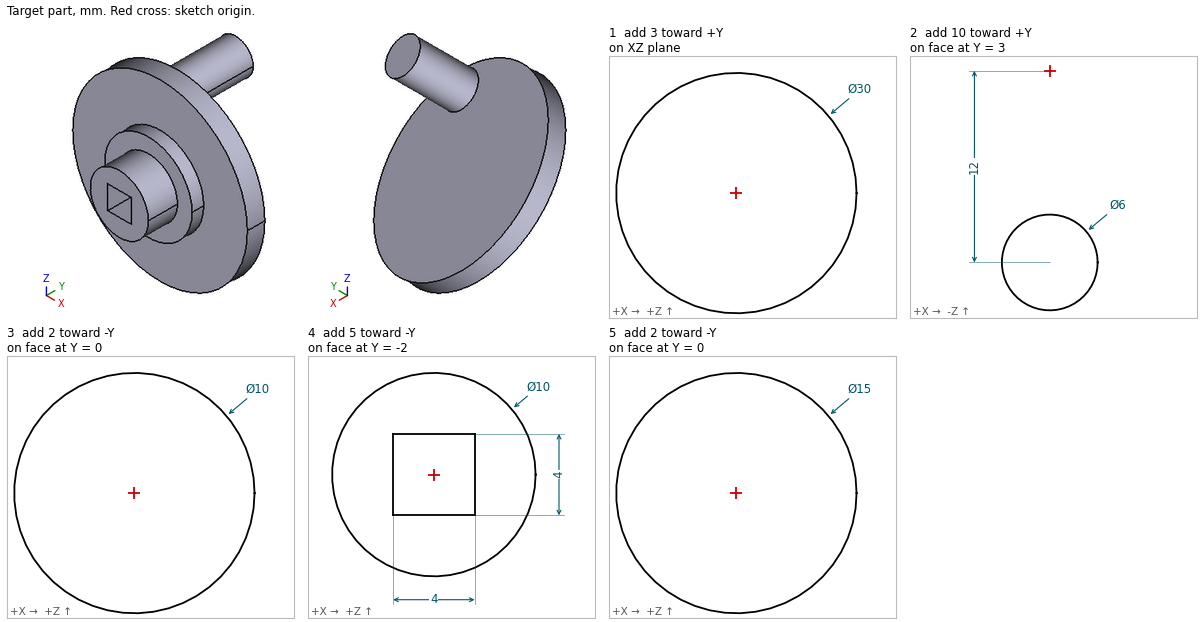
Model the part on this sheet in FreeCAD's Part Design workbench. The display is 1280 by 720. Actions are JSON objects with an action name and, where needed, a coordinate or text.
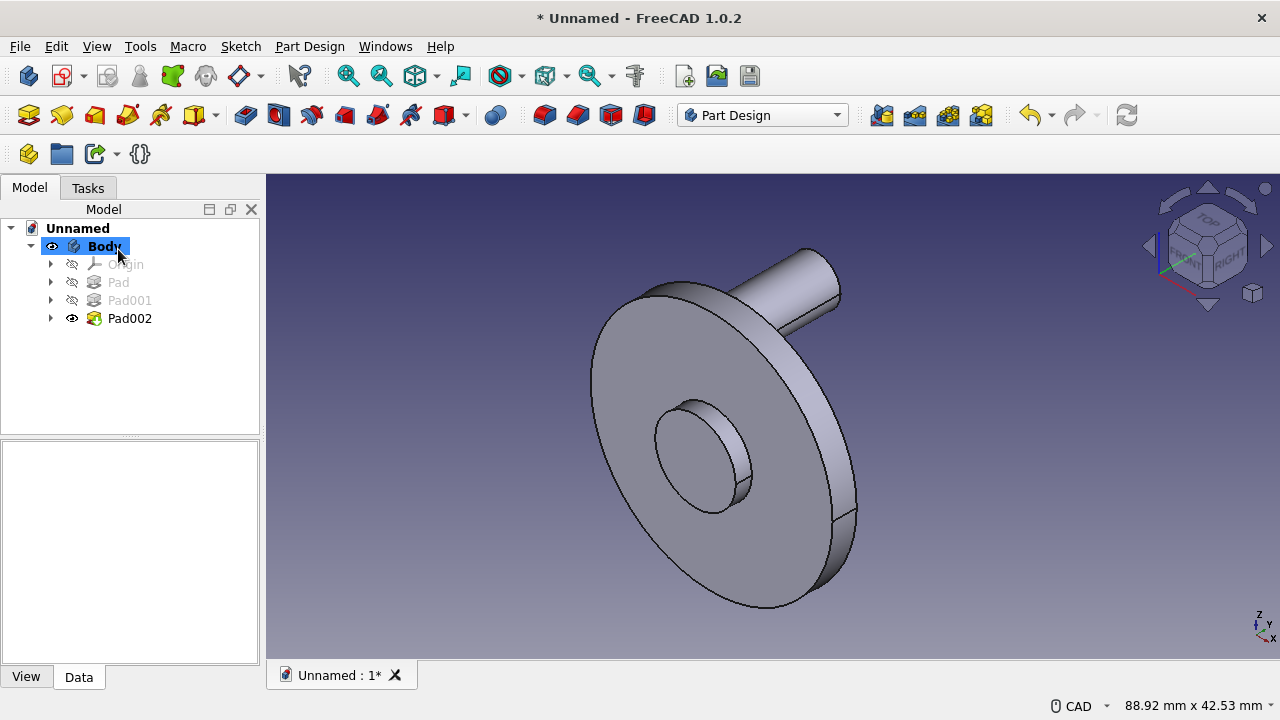
{"action": "left_click", "coordinate": [349, 76]}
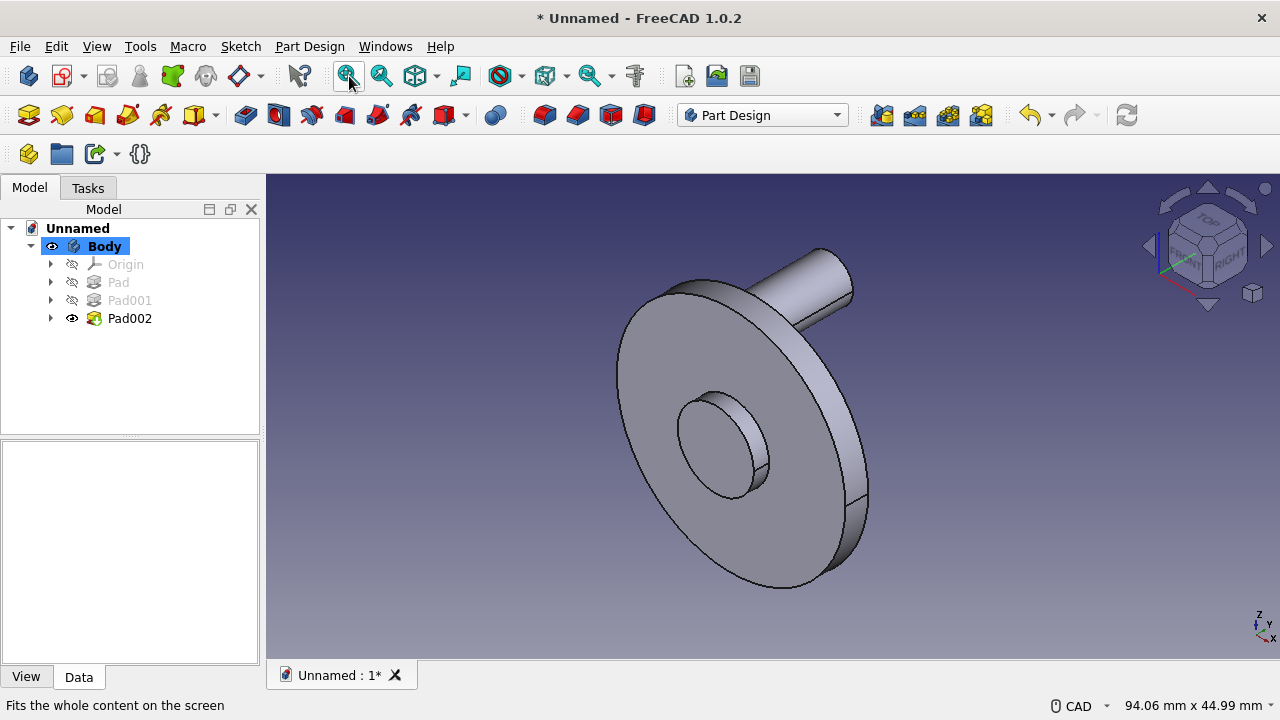
{"action": "left_click", "coordinate": [716, 449]}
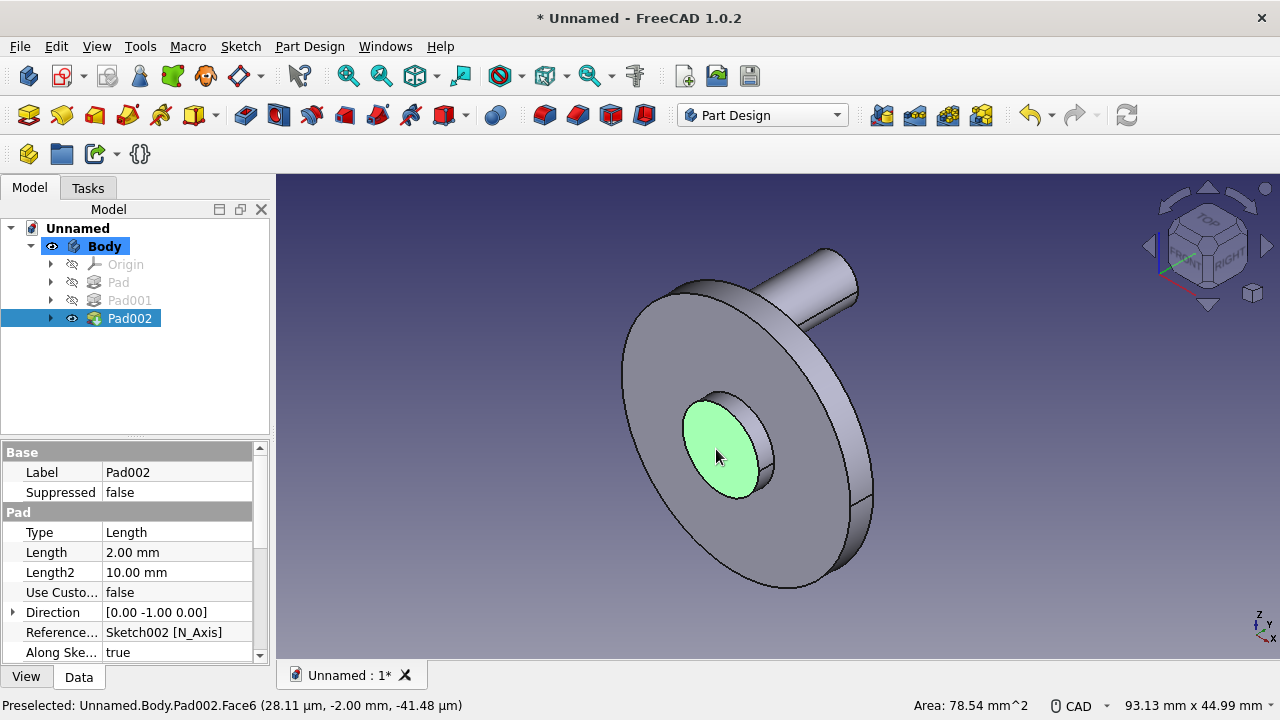
{"action": "left_click", "coordinate": [62, 76]}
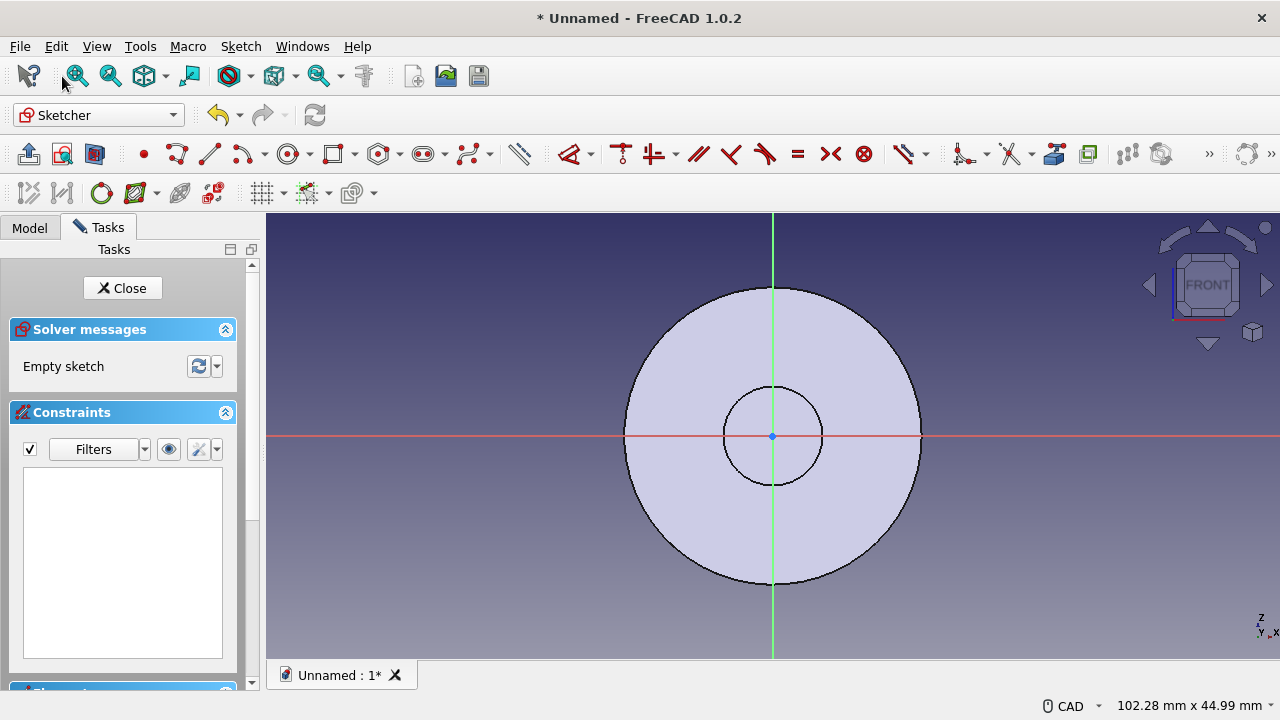
{"action": "scroll", "coordinate": [813, 436], "scroll_direction": "up", "scroll_amount": 5}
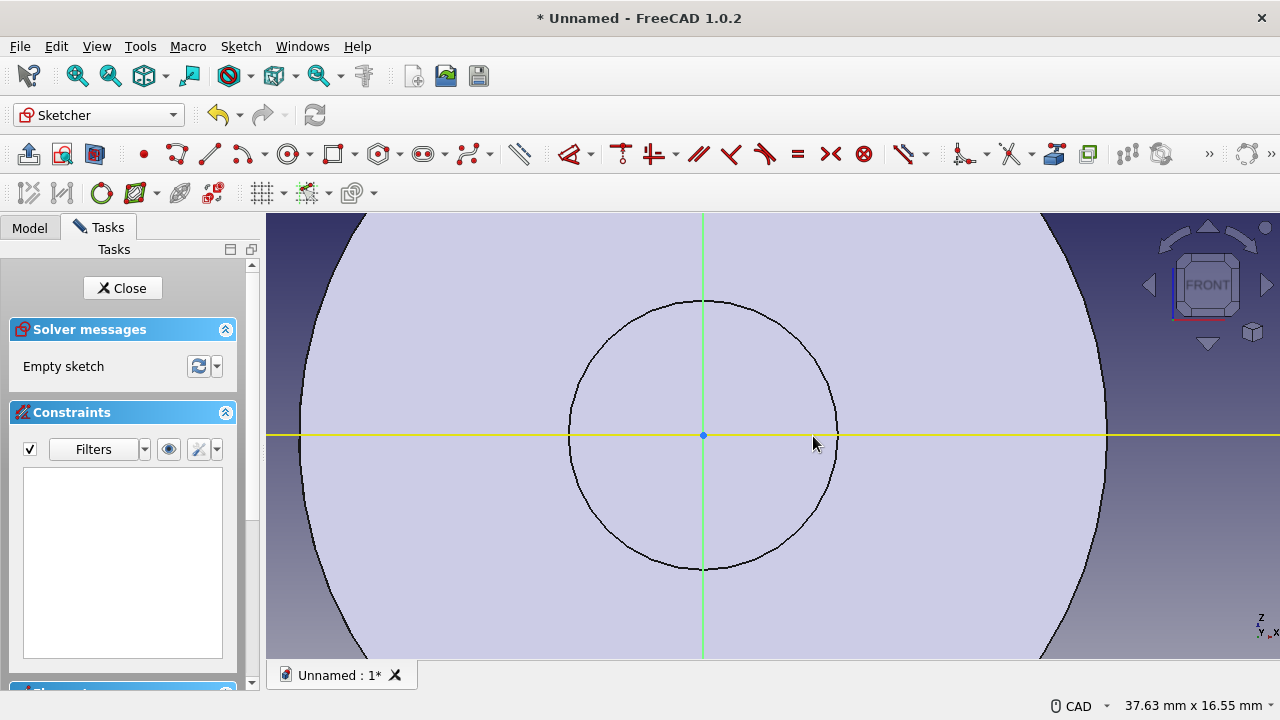
{"action": "left_click", "coordinate": [354, 154]}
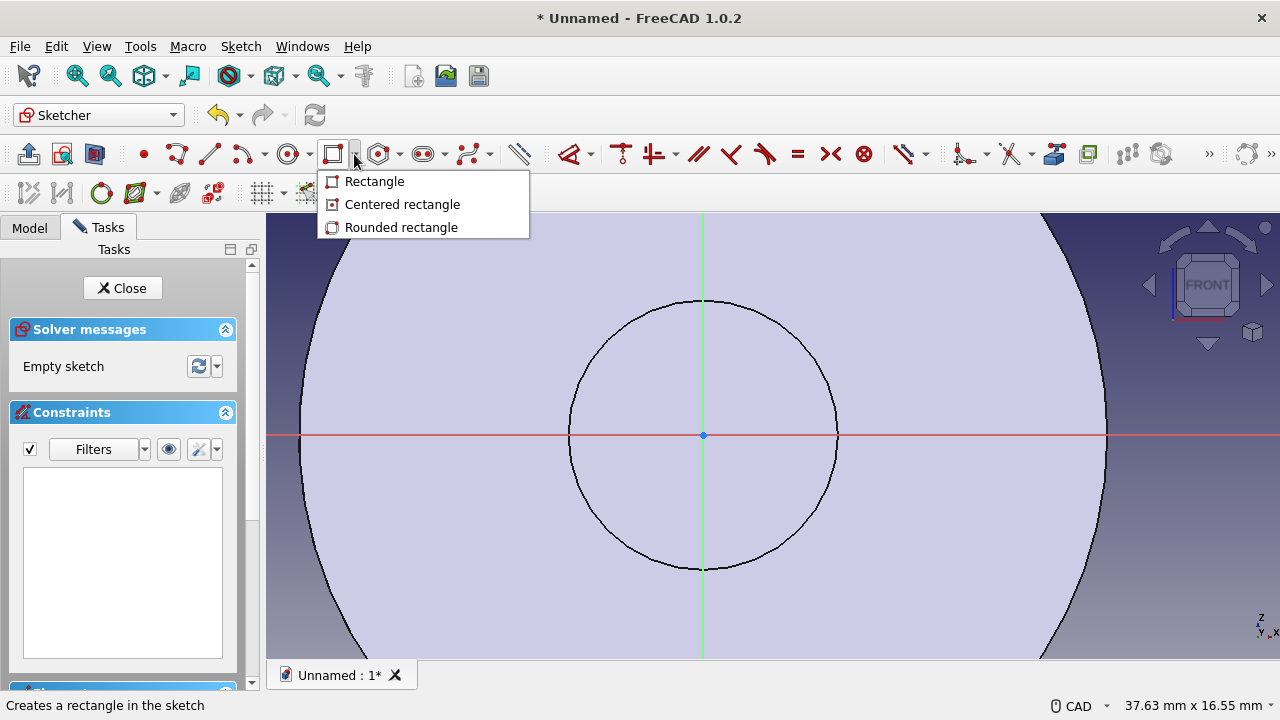
{"action": "left_click", "coordinate": [424, 204]}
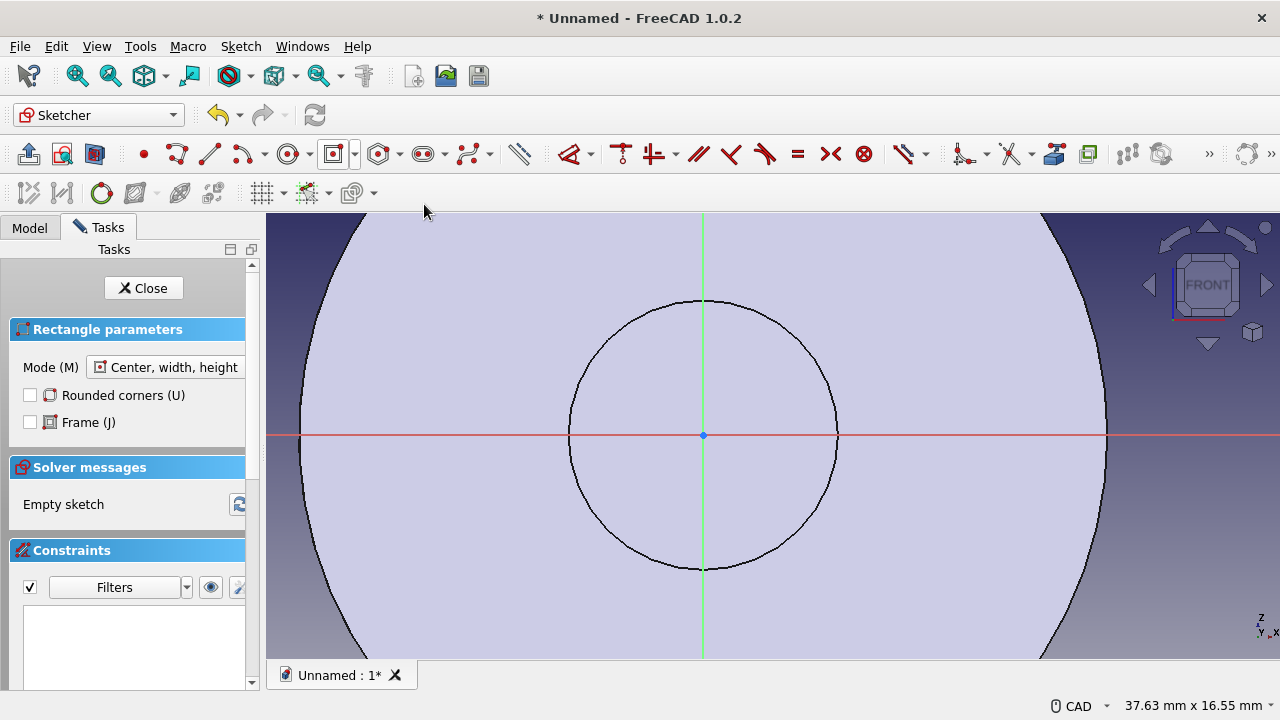
{"action": "left_click", "coordinate": [703, 435]}
{"action": "left_click", "coordinate": [757, 381]}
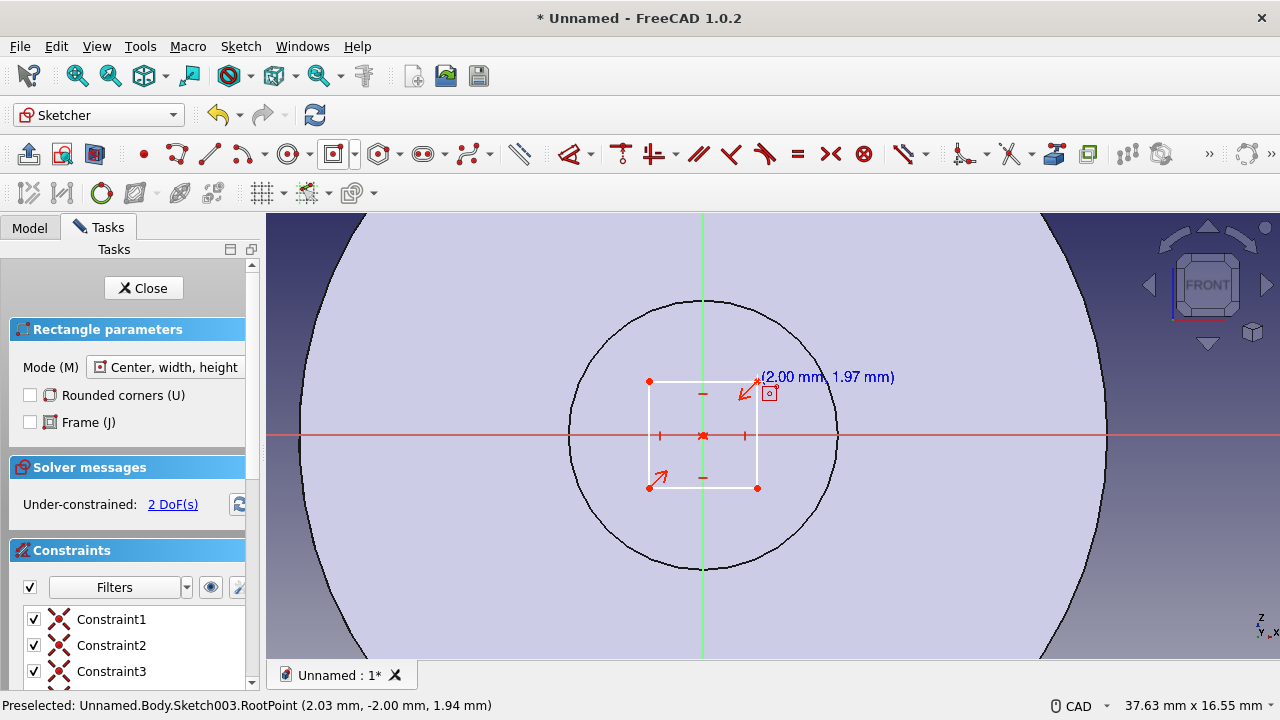
{"action": "left_click", "coordinate": [288, 154]}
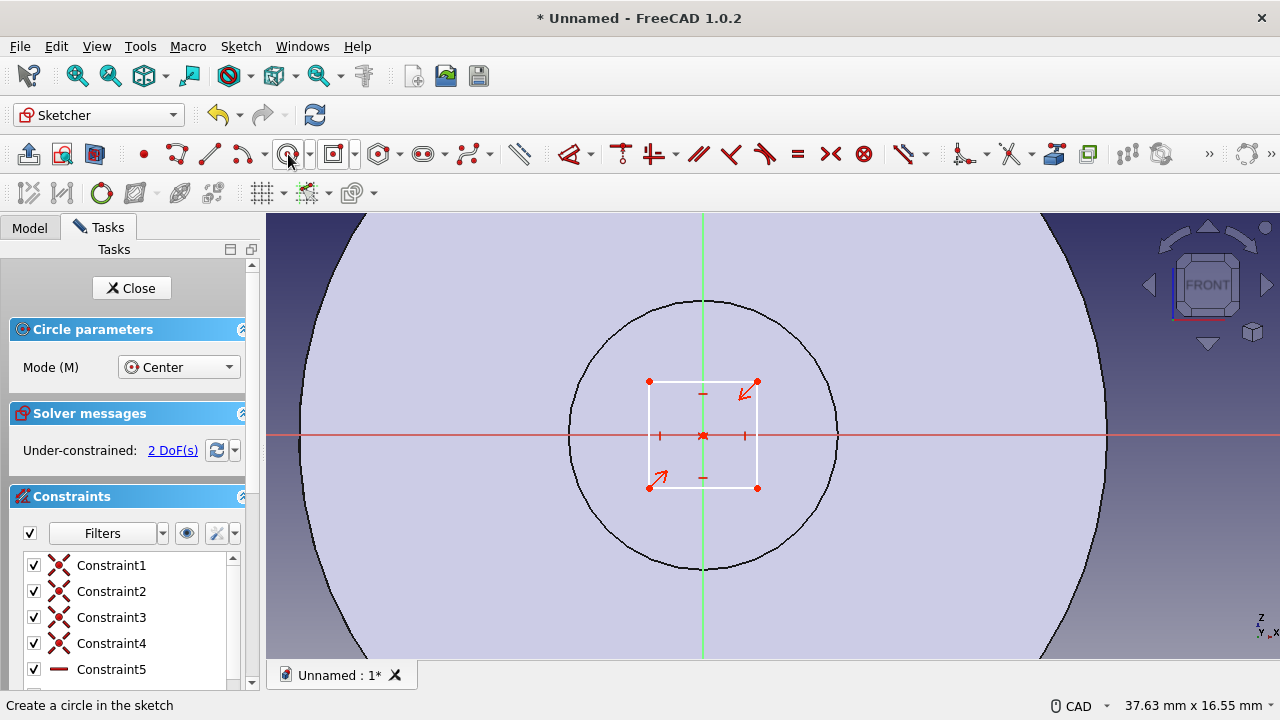
{"action": "left_click", "coordinate": [703, 435]}
{"action": "left_click", "coordinate": [798, 340]}
{"action": "key", "text": "Escape"}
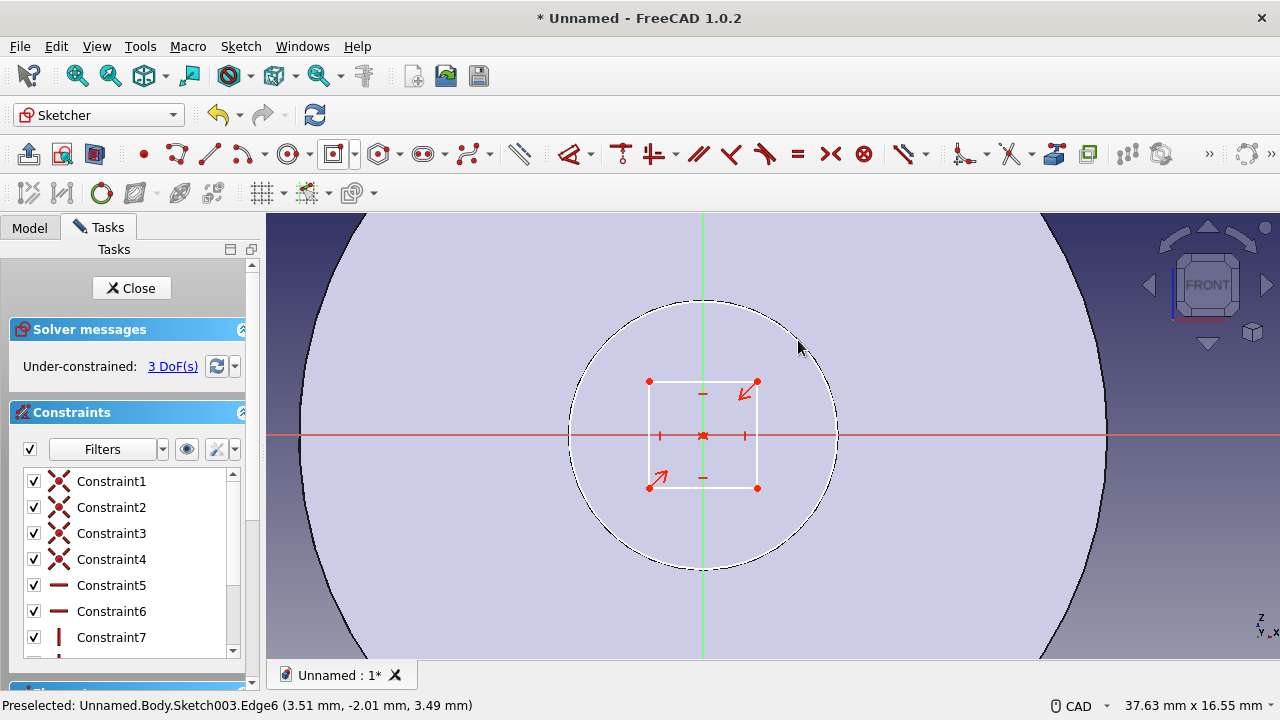
{"action": "left_click", "coordinate": [568, 154]}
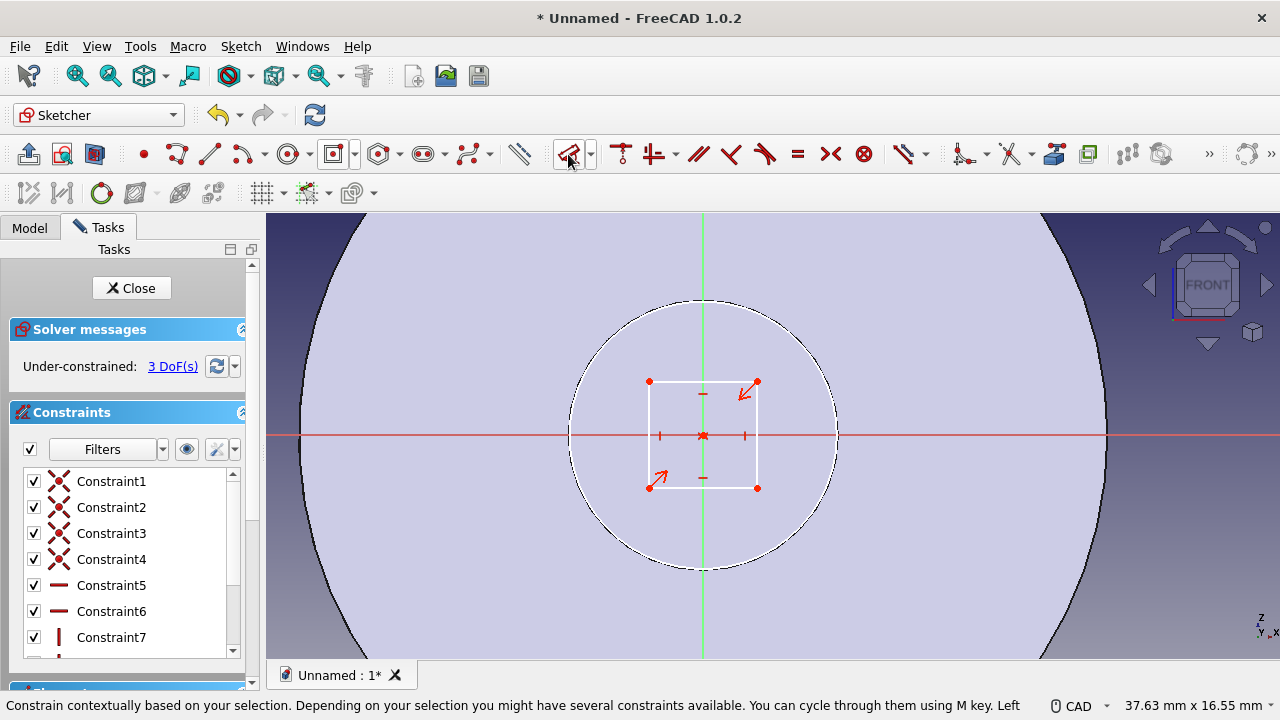
{"action": "left_click", "coordinate": [797, 340]}
{"action": "left_click", "coordinate": [819, 317]}